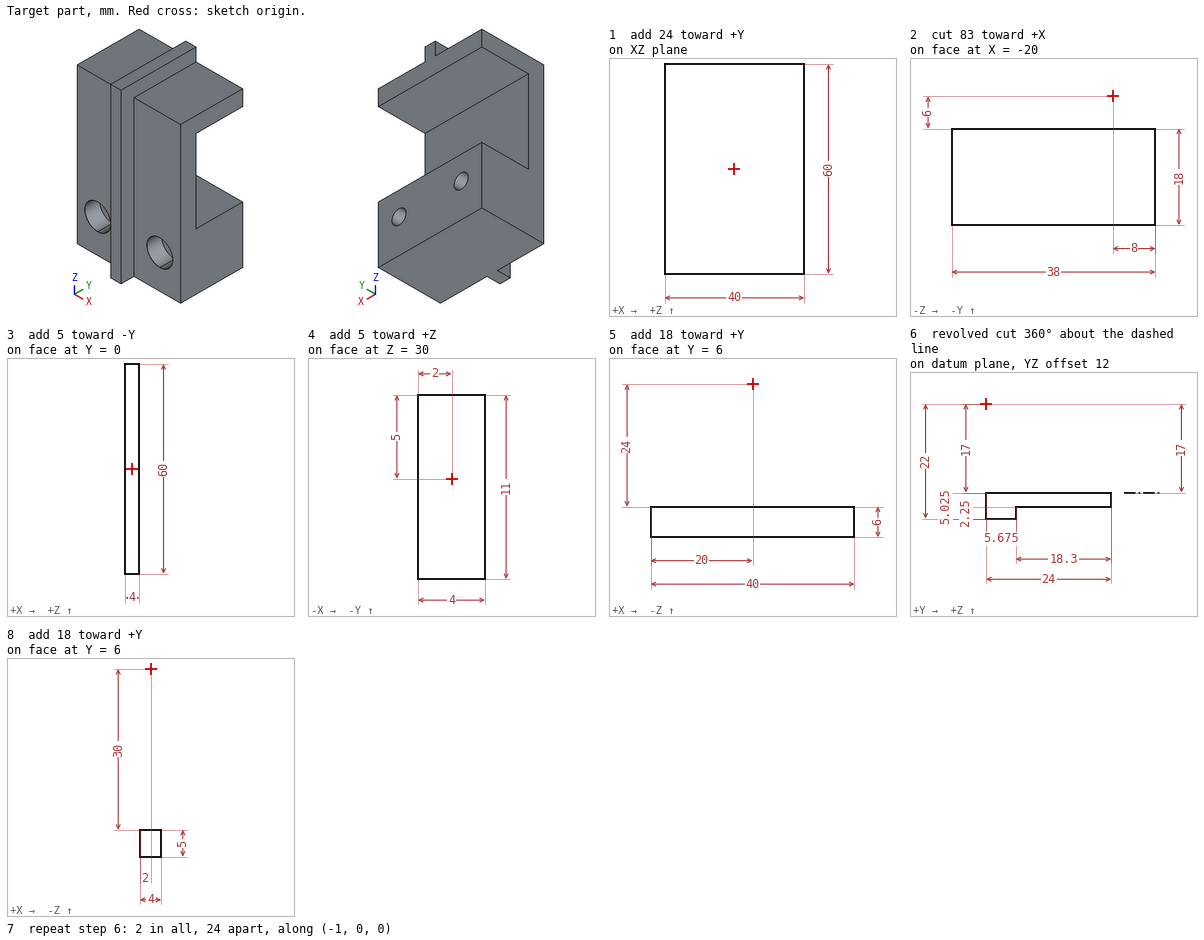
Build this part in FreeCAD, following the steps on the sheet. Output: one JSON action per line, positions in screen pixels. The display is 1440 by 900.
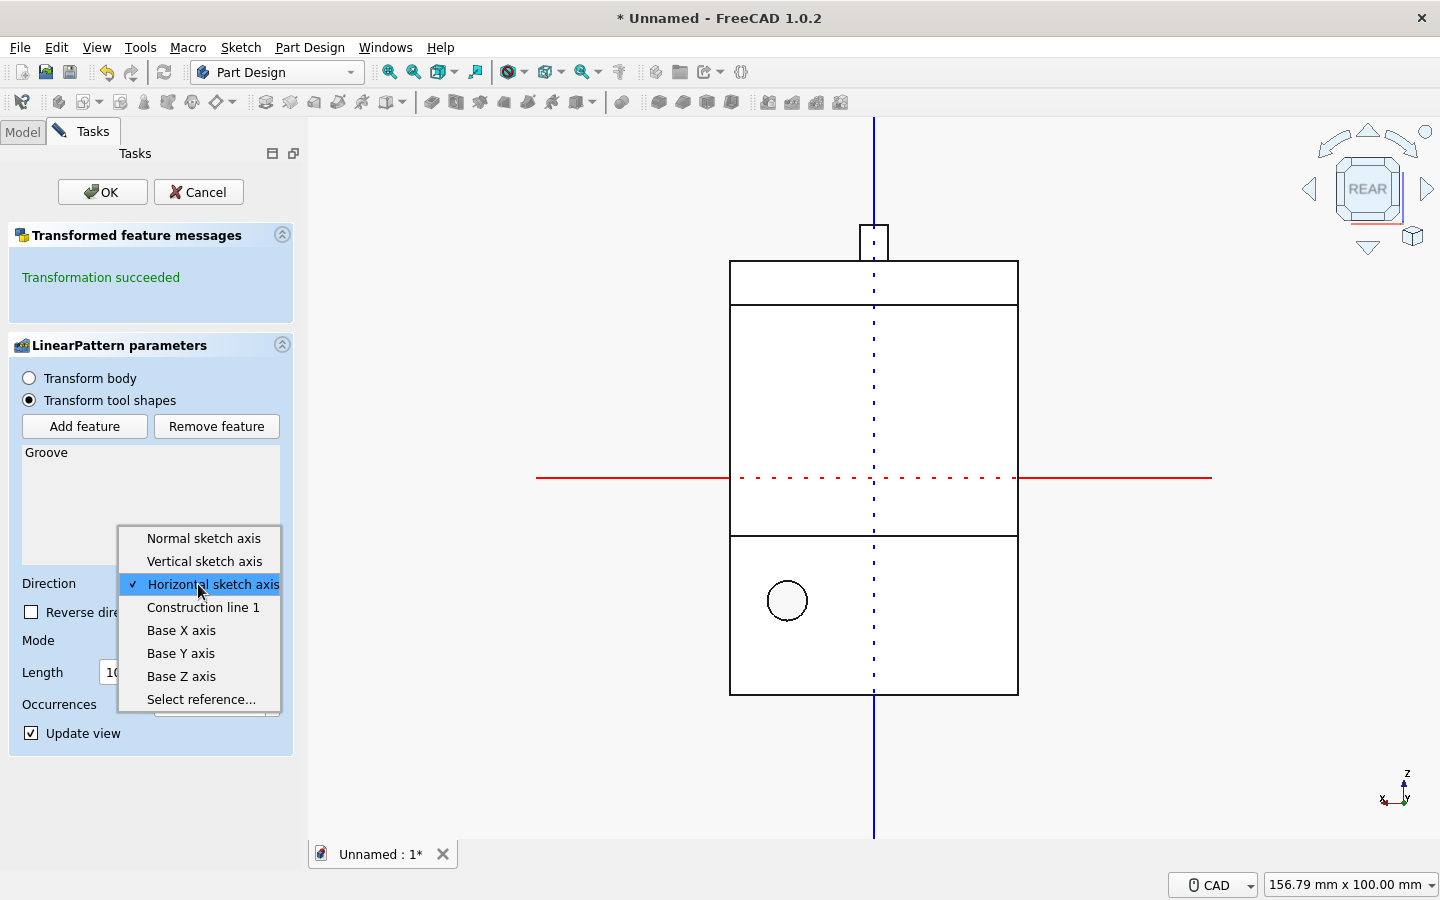
{"action": "left_click", "coordinate": [198, 630]}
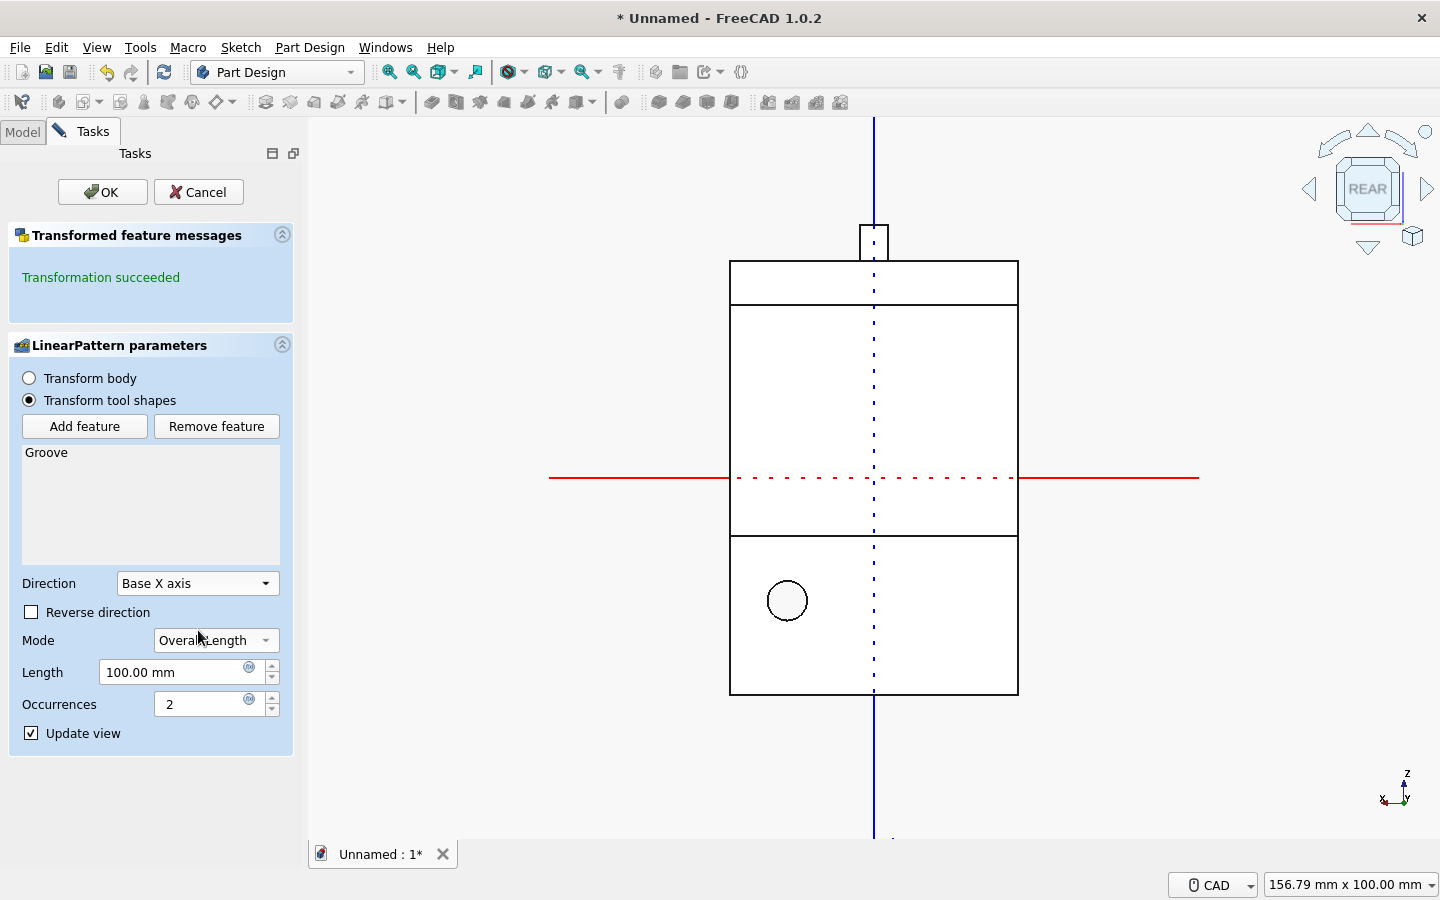
{"action": "left_click", "coordinate": [217, 640]}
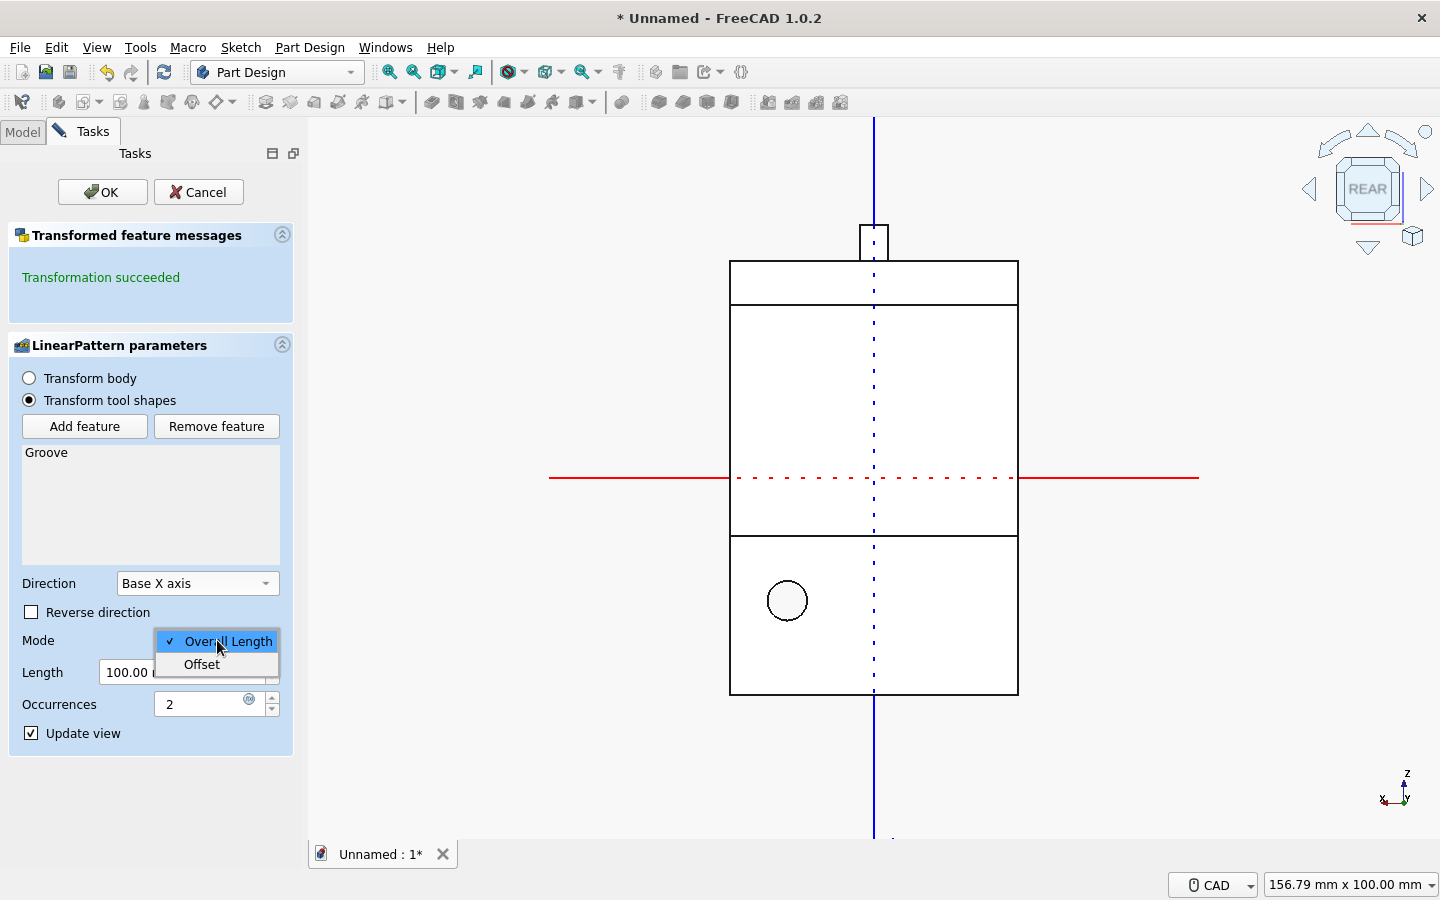
{"action": "left_click", "coordinate": [216, 664]}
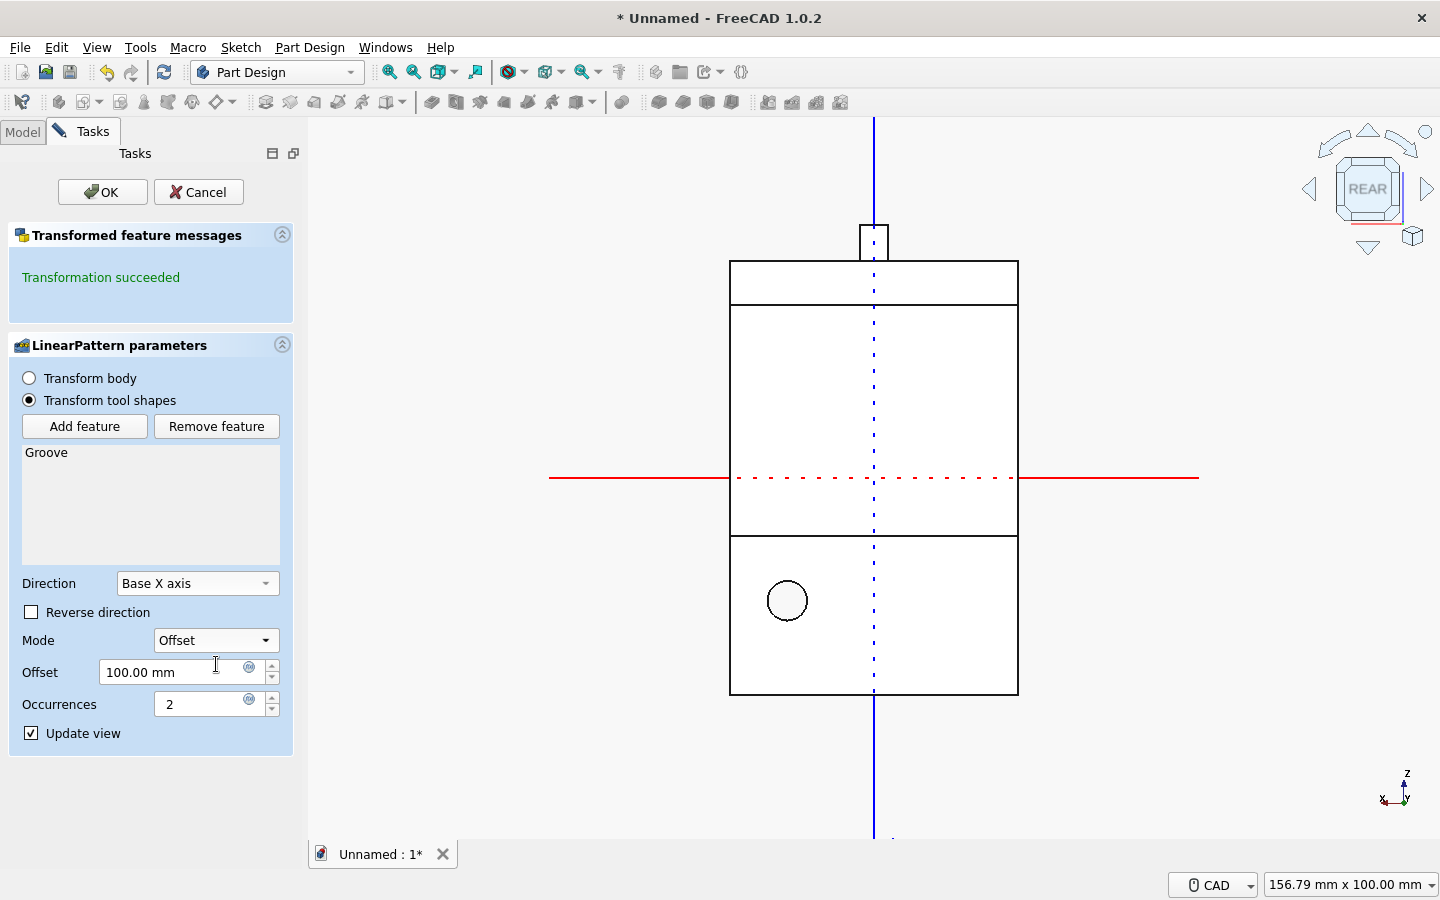
{"action": "triple_click", "coordinate": [182, 672]}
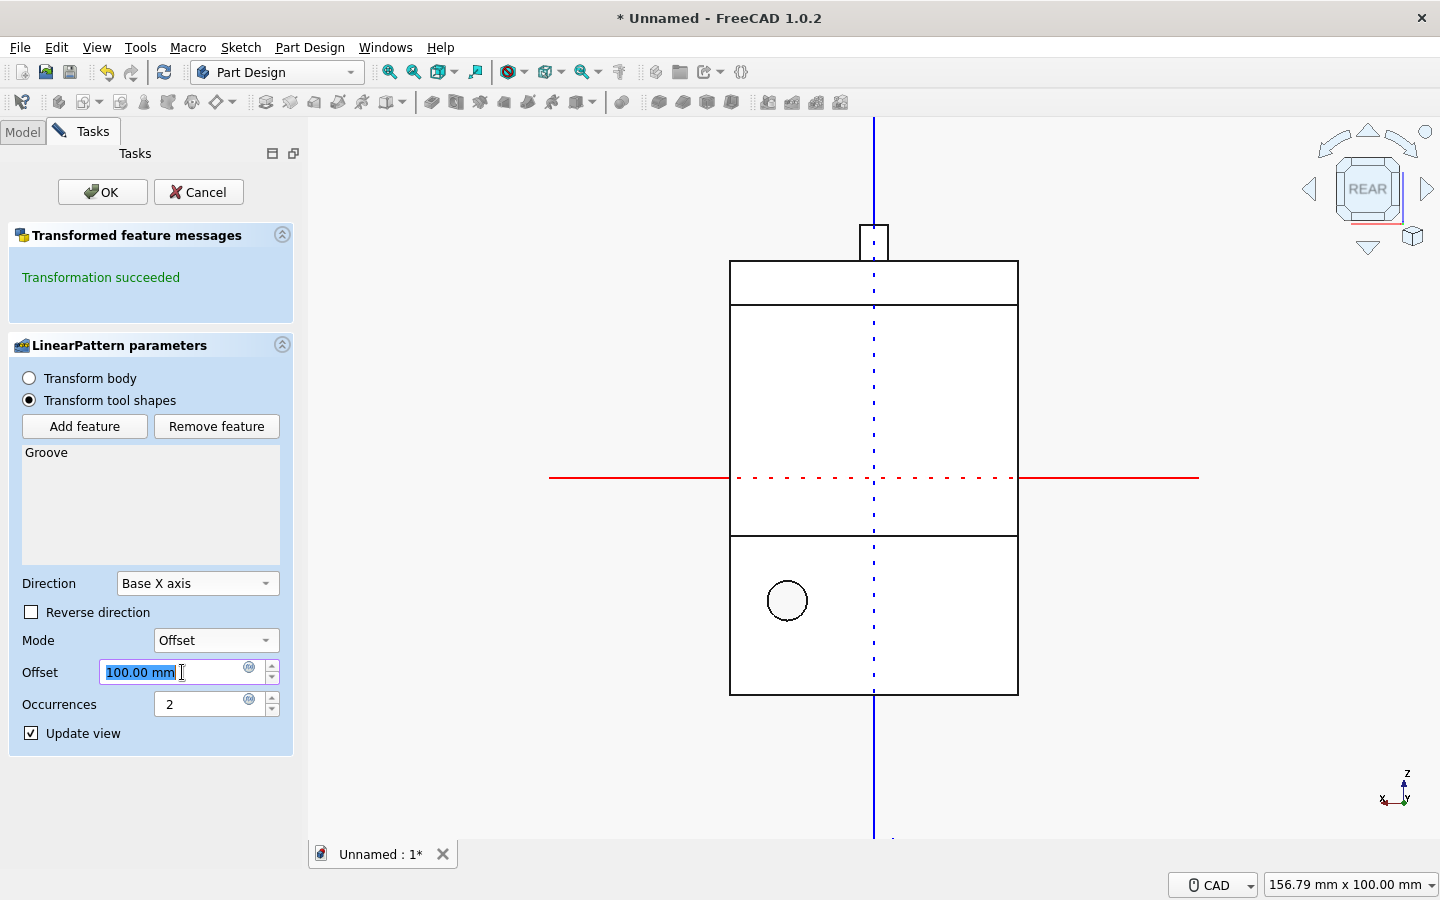
{"action": "type", "text": "24"}
{"action": "key", "text": "Tab"}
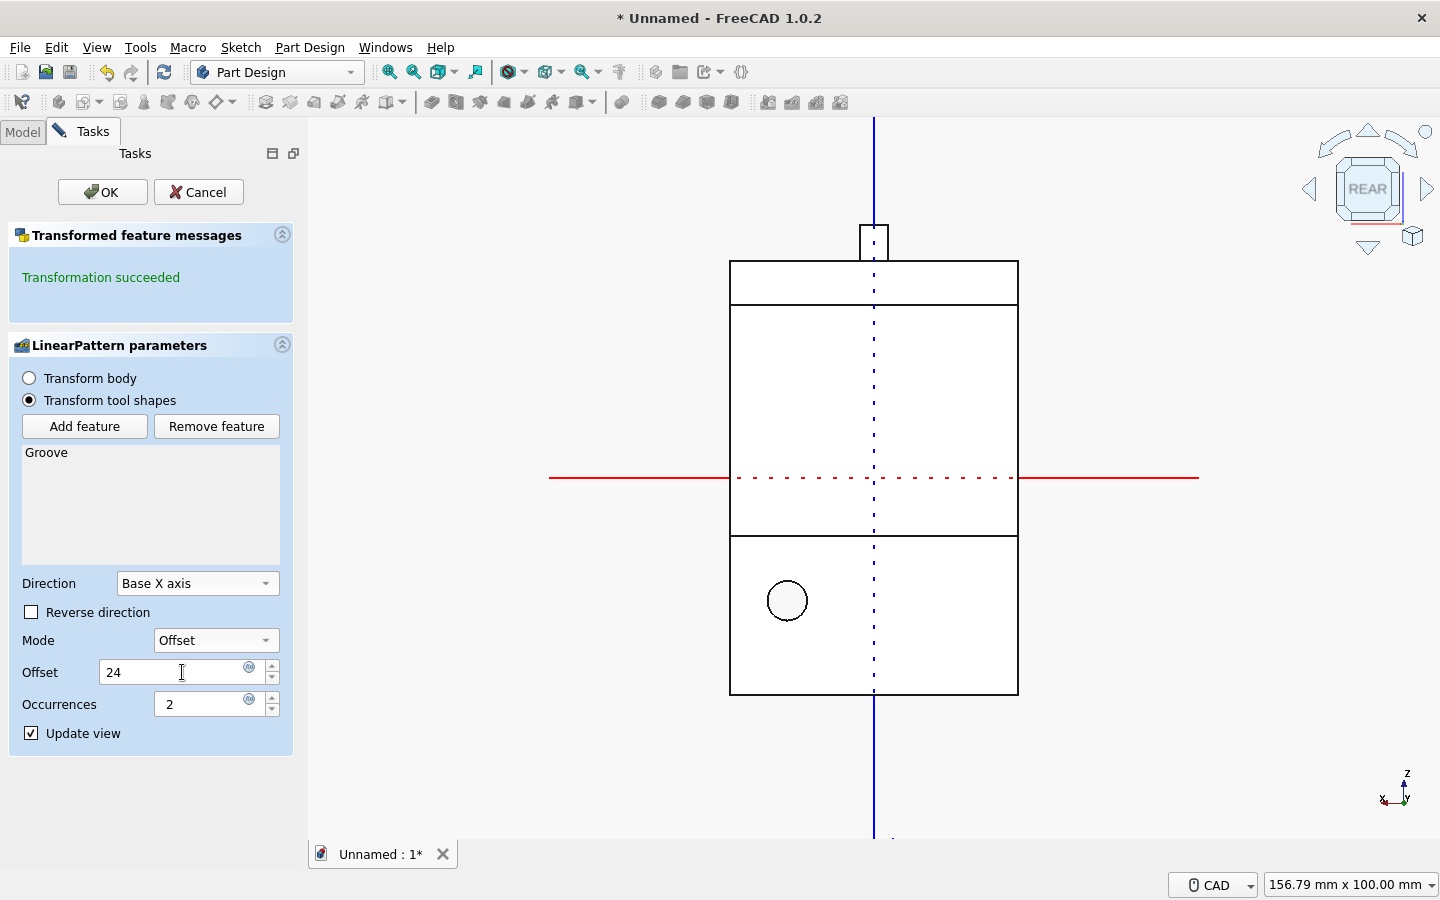
{"action": "triple_click", "coordinate": [209, 704]}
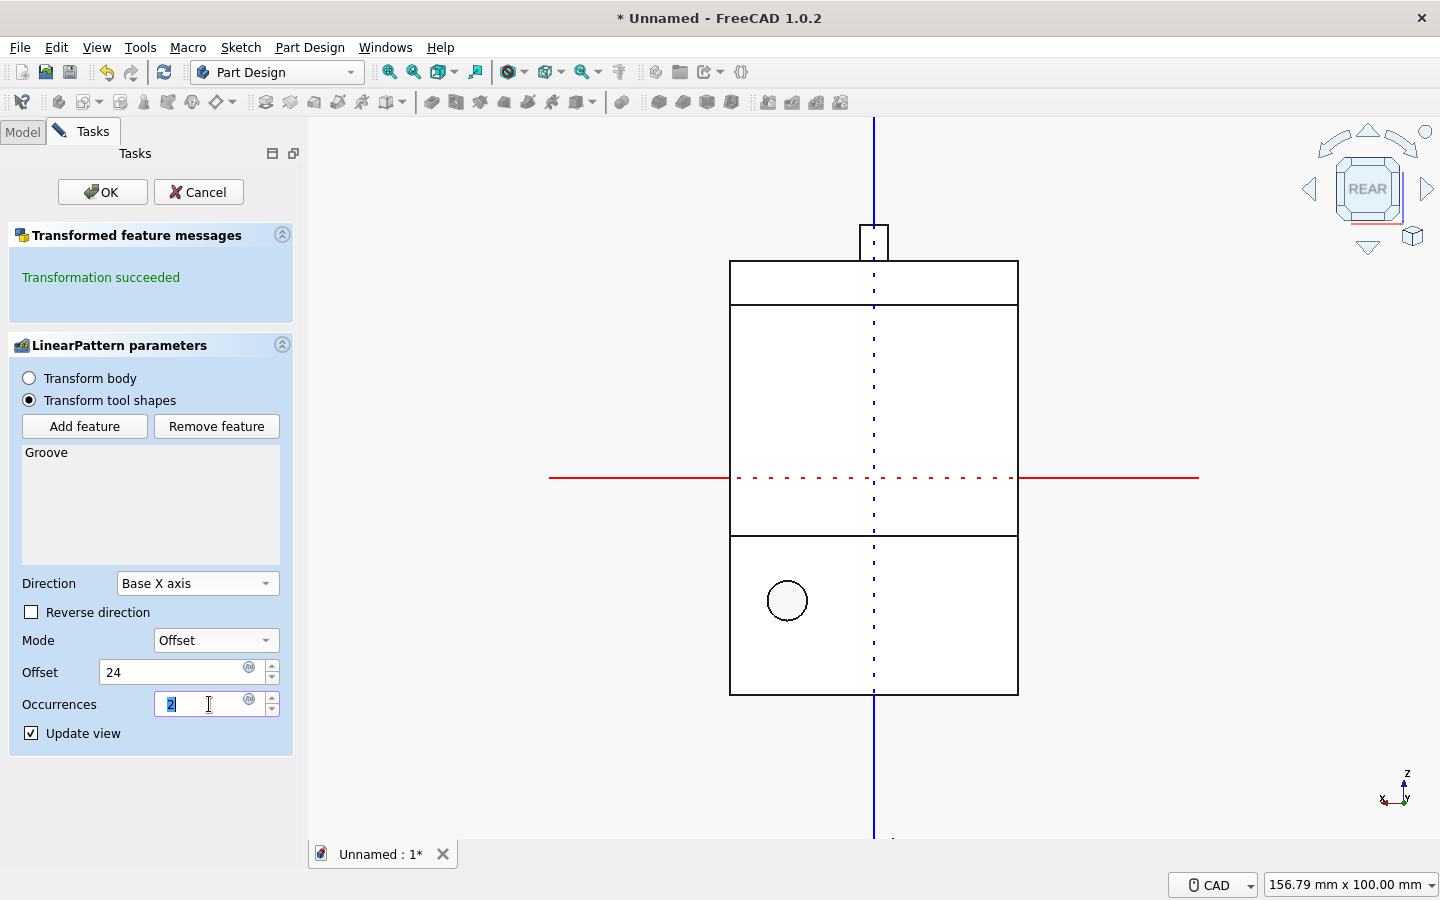
{"action": "type", "text": "2"}
{"action": "key", "text": "Tab"}